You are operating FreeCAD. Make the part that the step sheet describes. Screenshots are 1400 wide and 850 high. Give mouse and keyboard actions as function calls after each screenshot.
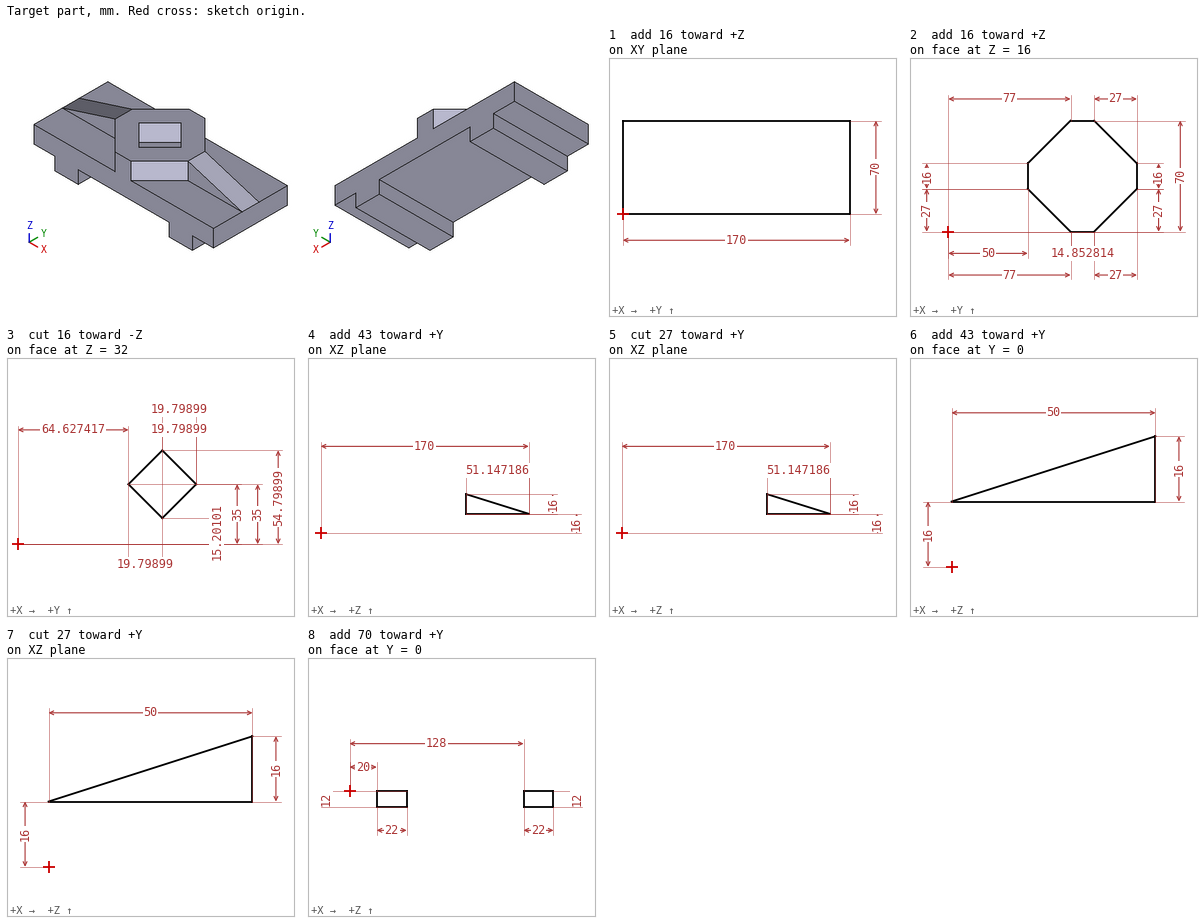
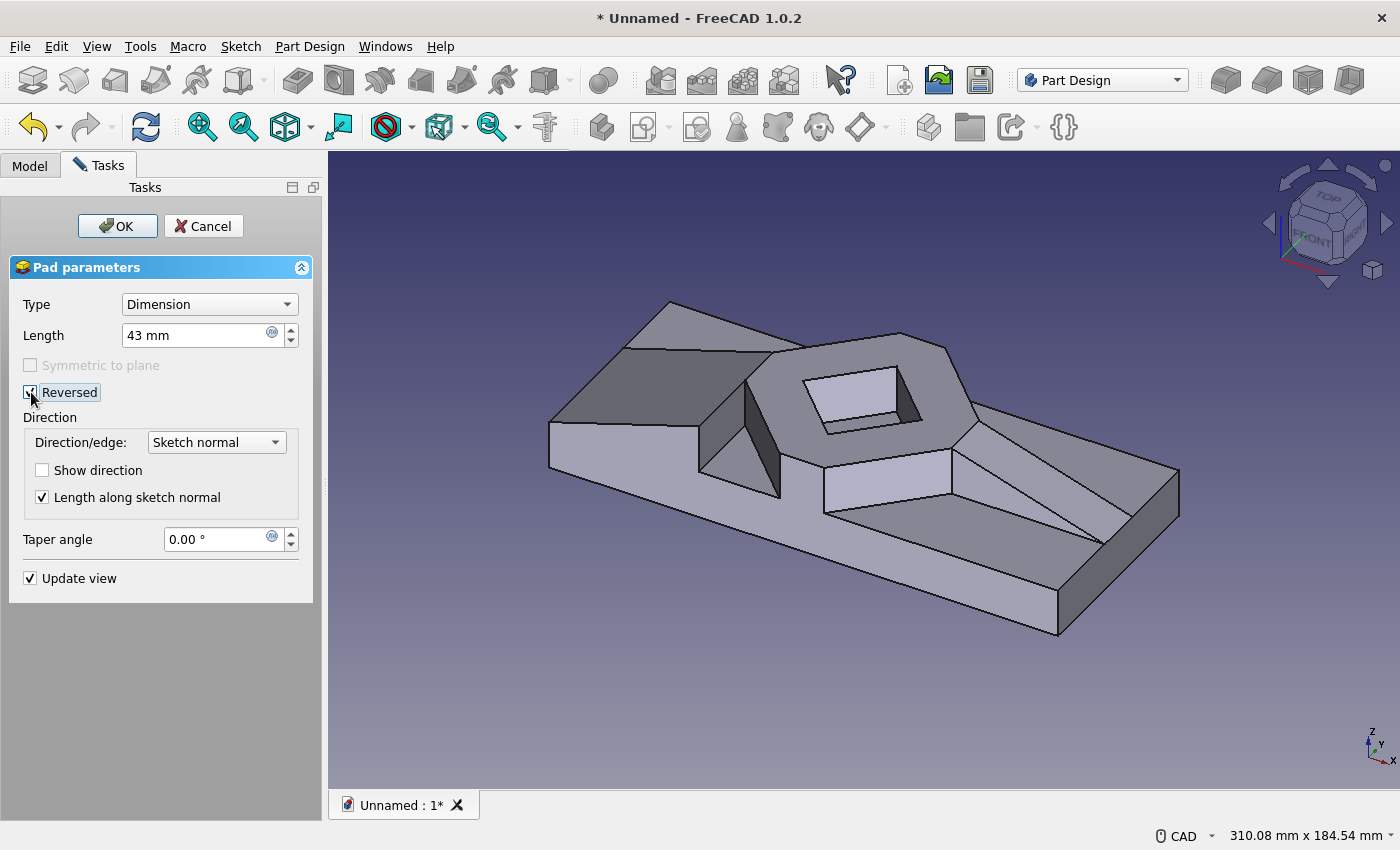
click(118, 226)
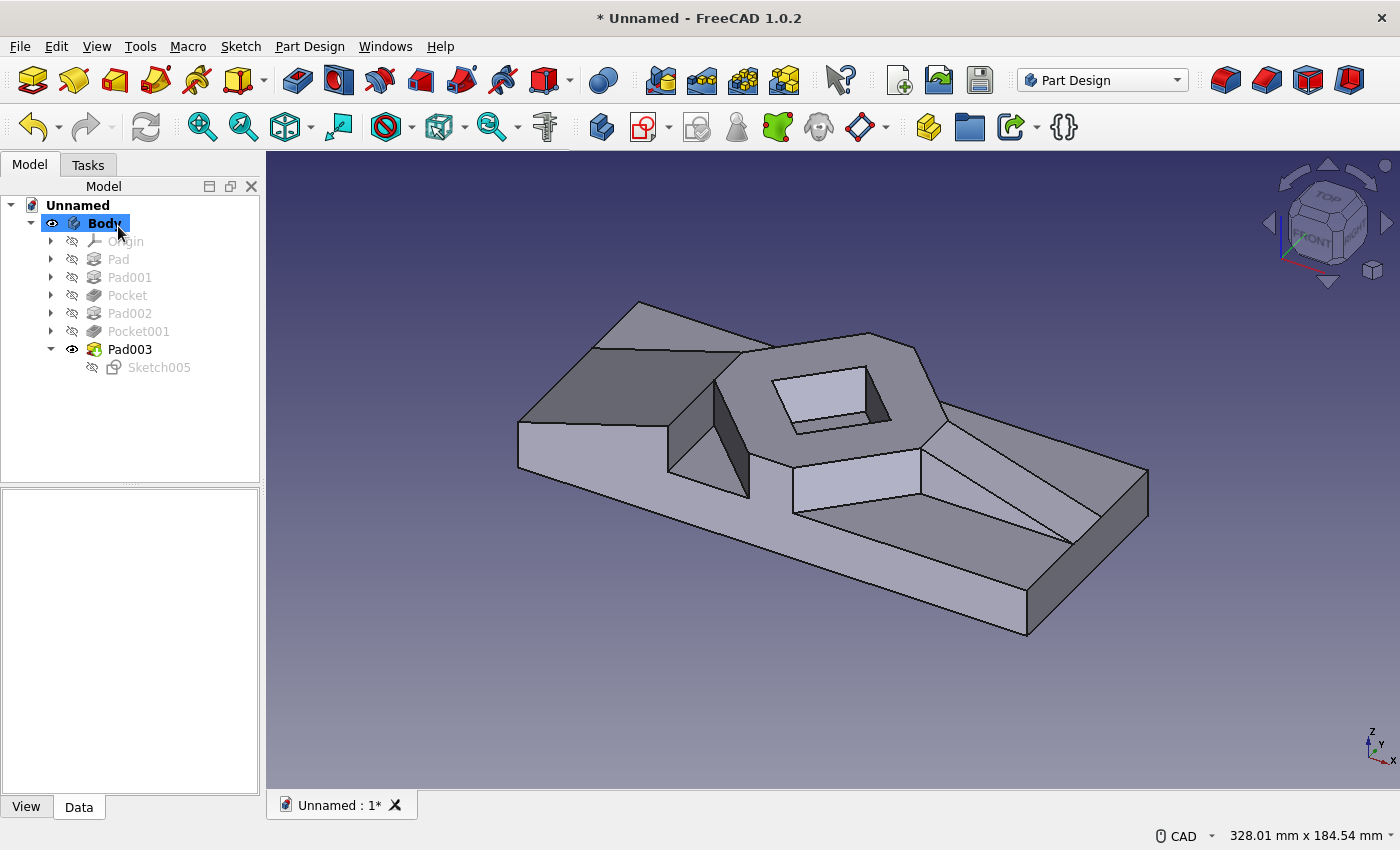
click(642, 128)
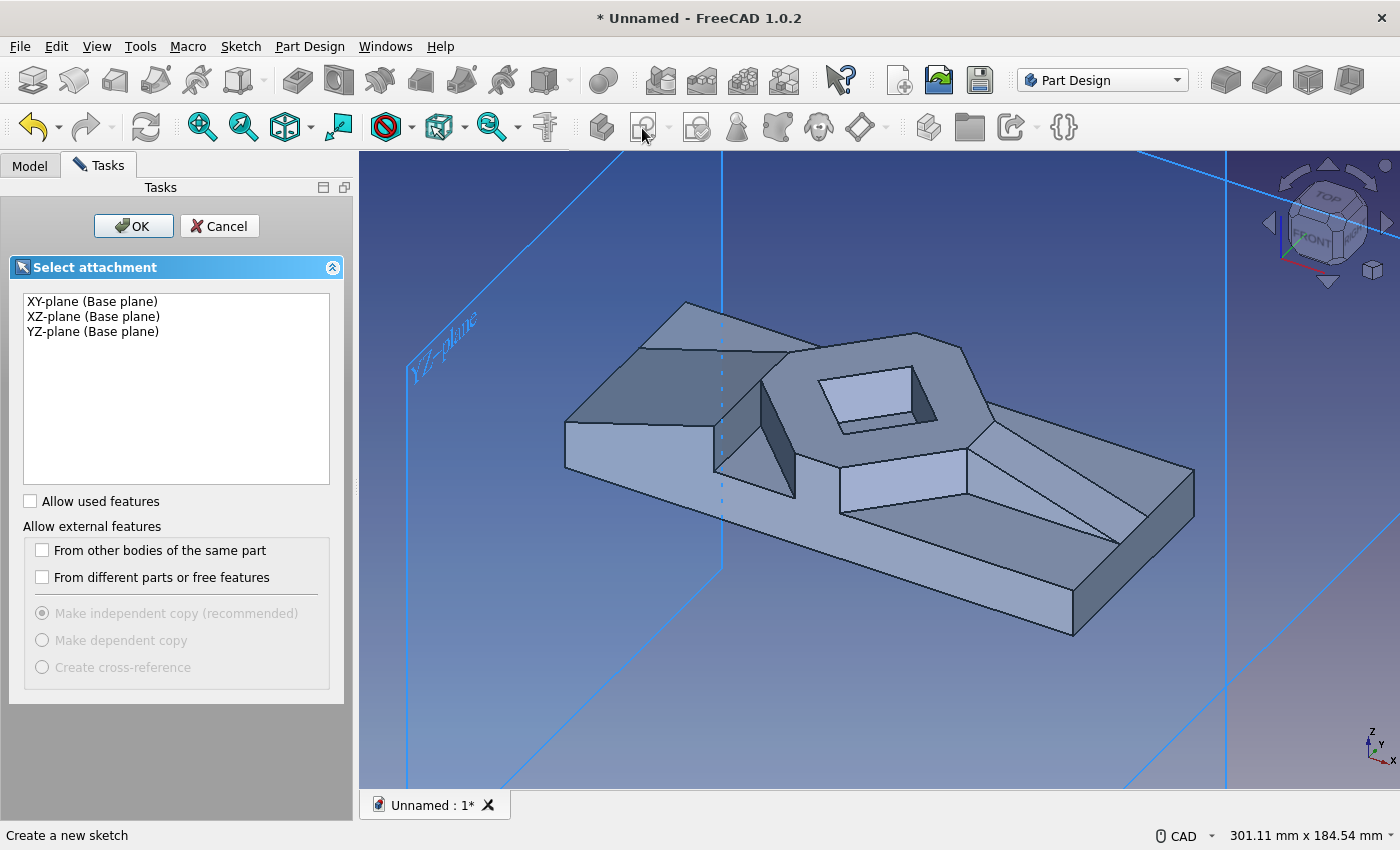
click(84, 316)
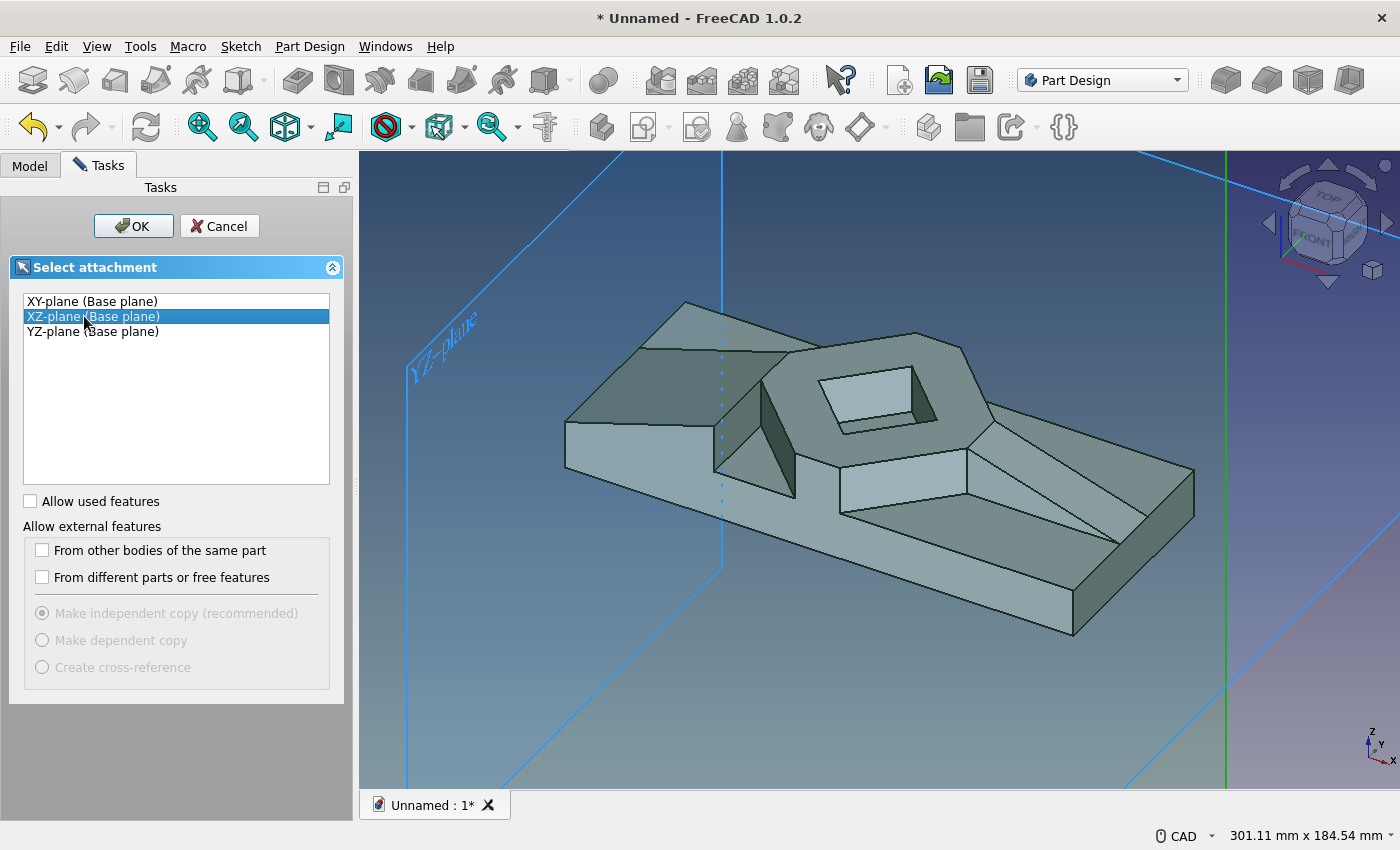
click(134, 226)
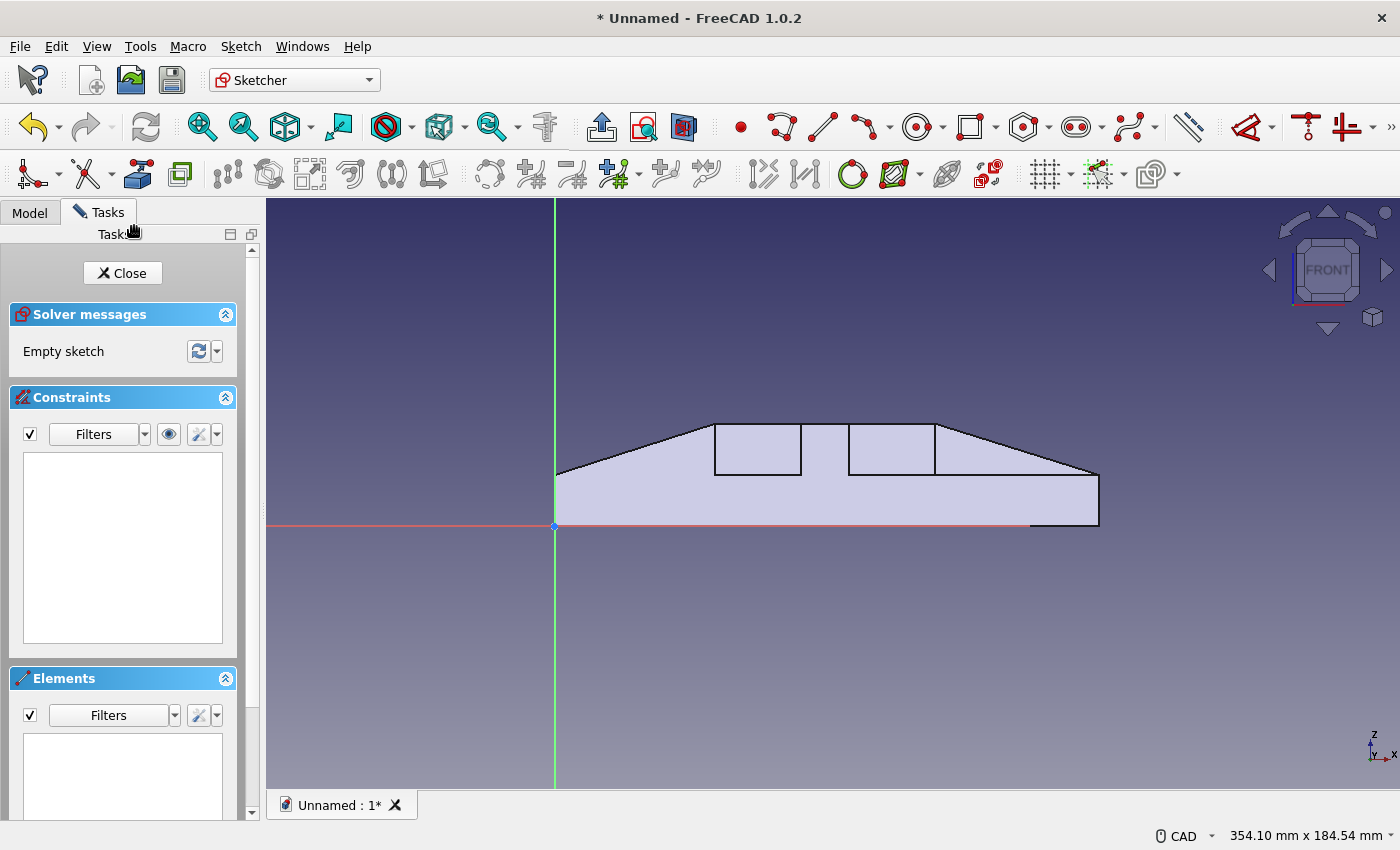
scroll(592, 469, up, 7)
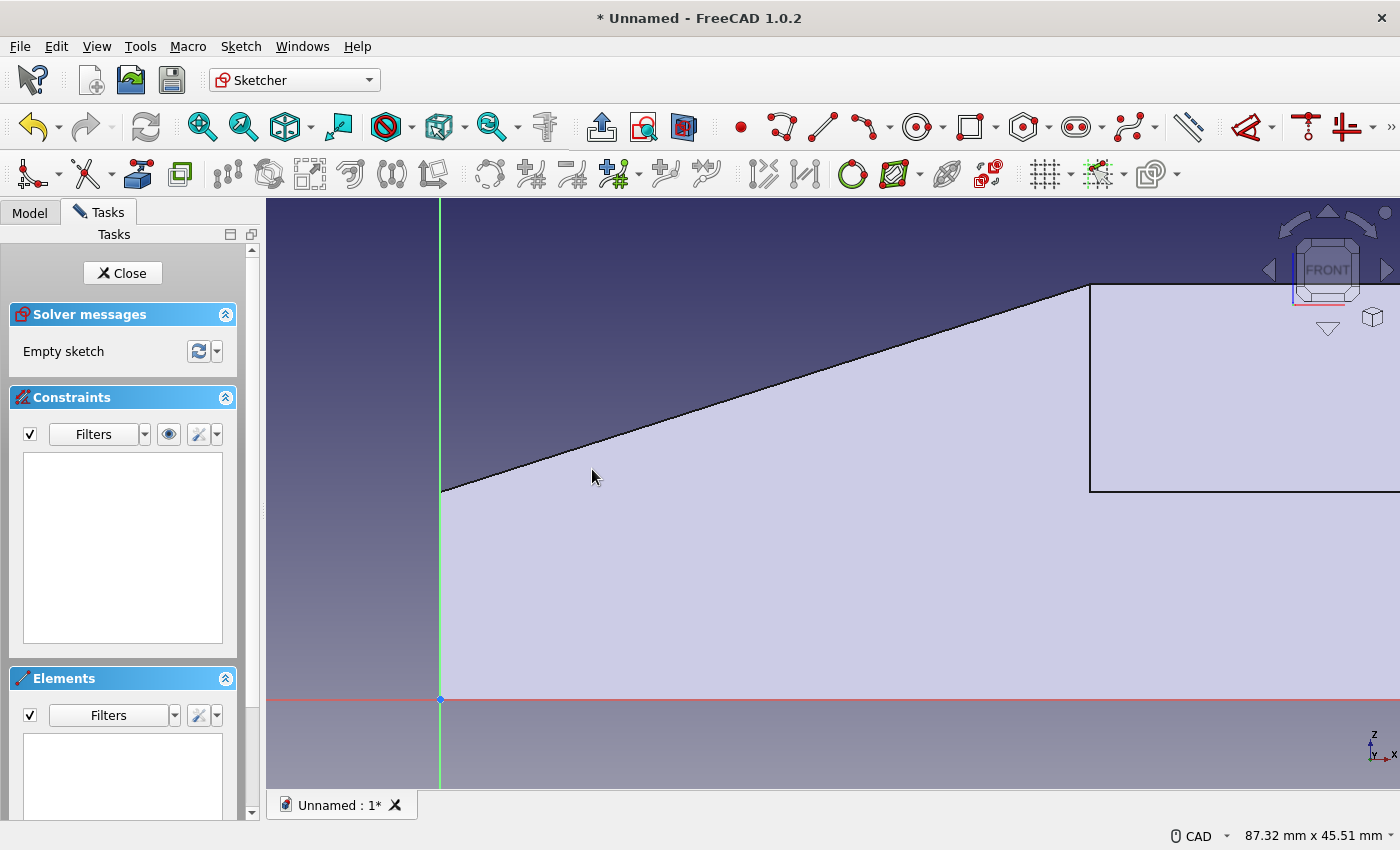
key(g)
key(m)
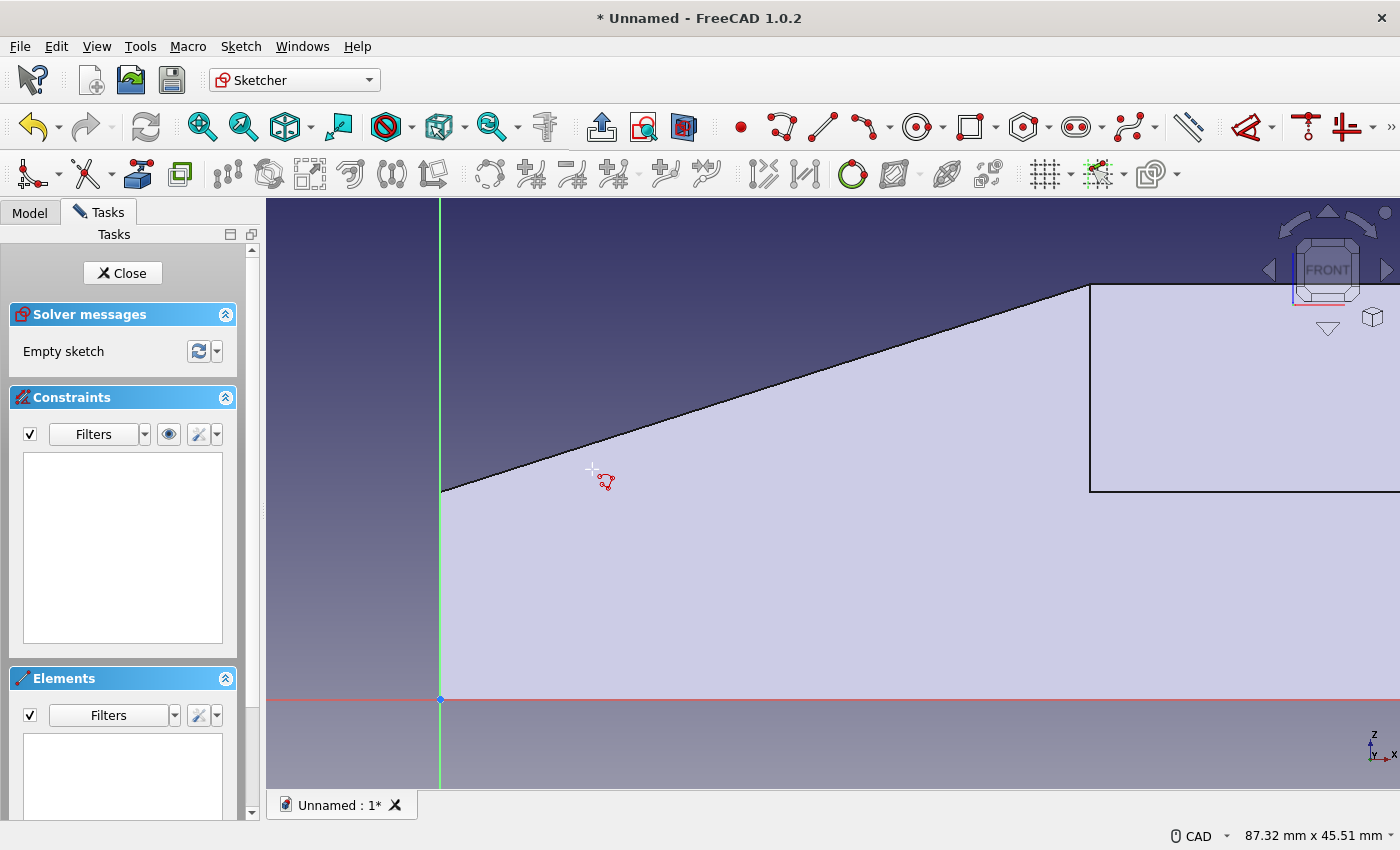
click(440, 492)
click(1090, 492)
click(1090, 284)
click(440, 493)
key(Escape)
key(Escape)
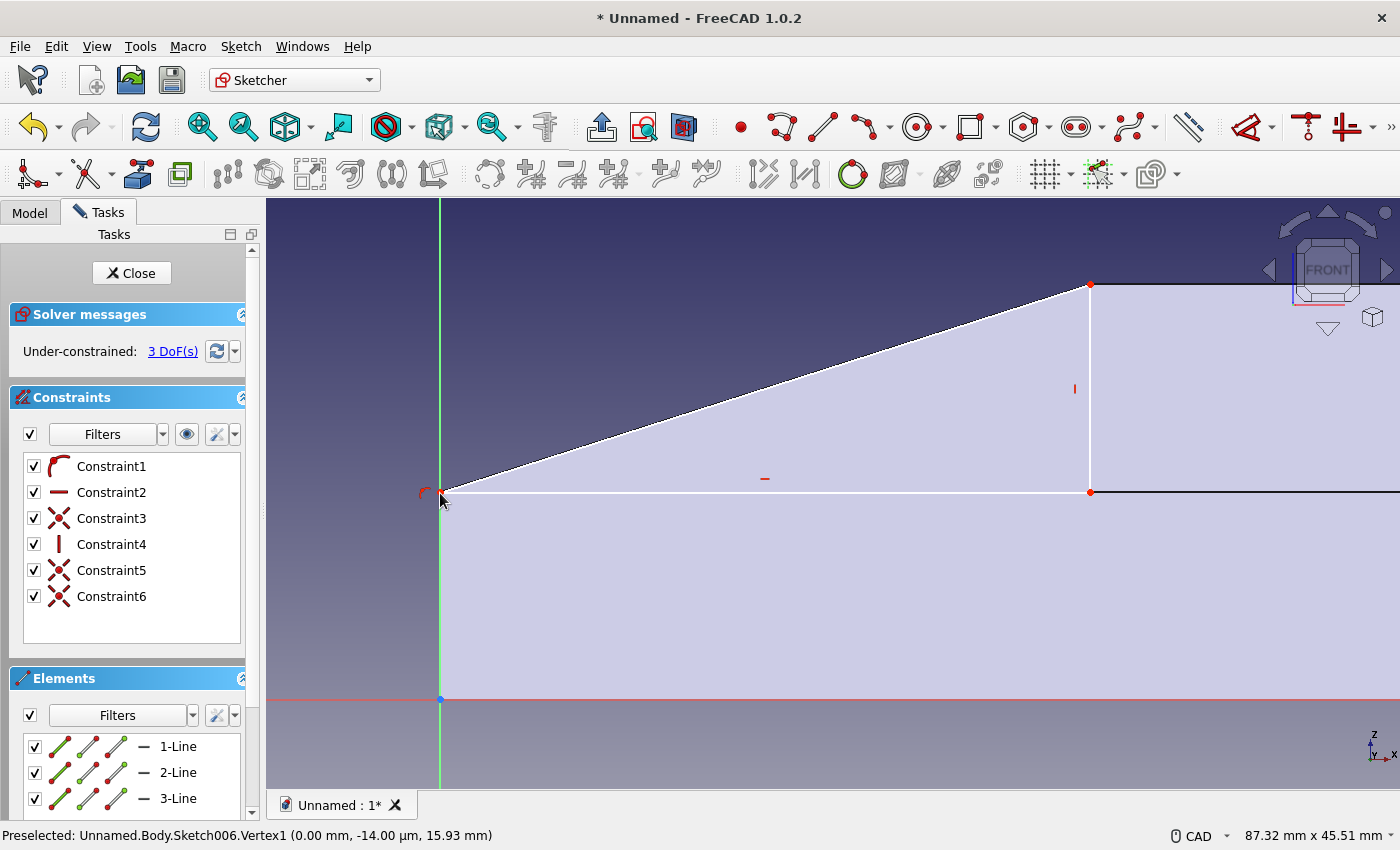
click(1246, 128)